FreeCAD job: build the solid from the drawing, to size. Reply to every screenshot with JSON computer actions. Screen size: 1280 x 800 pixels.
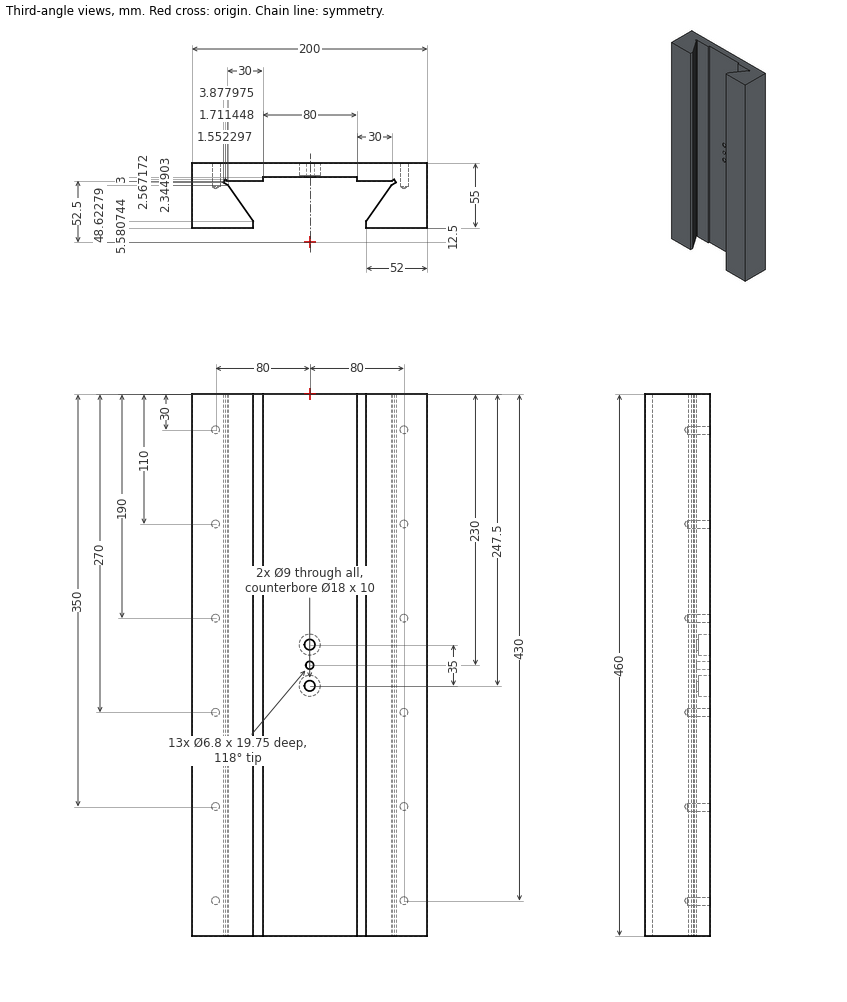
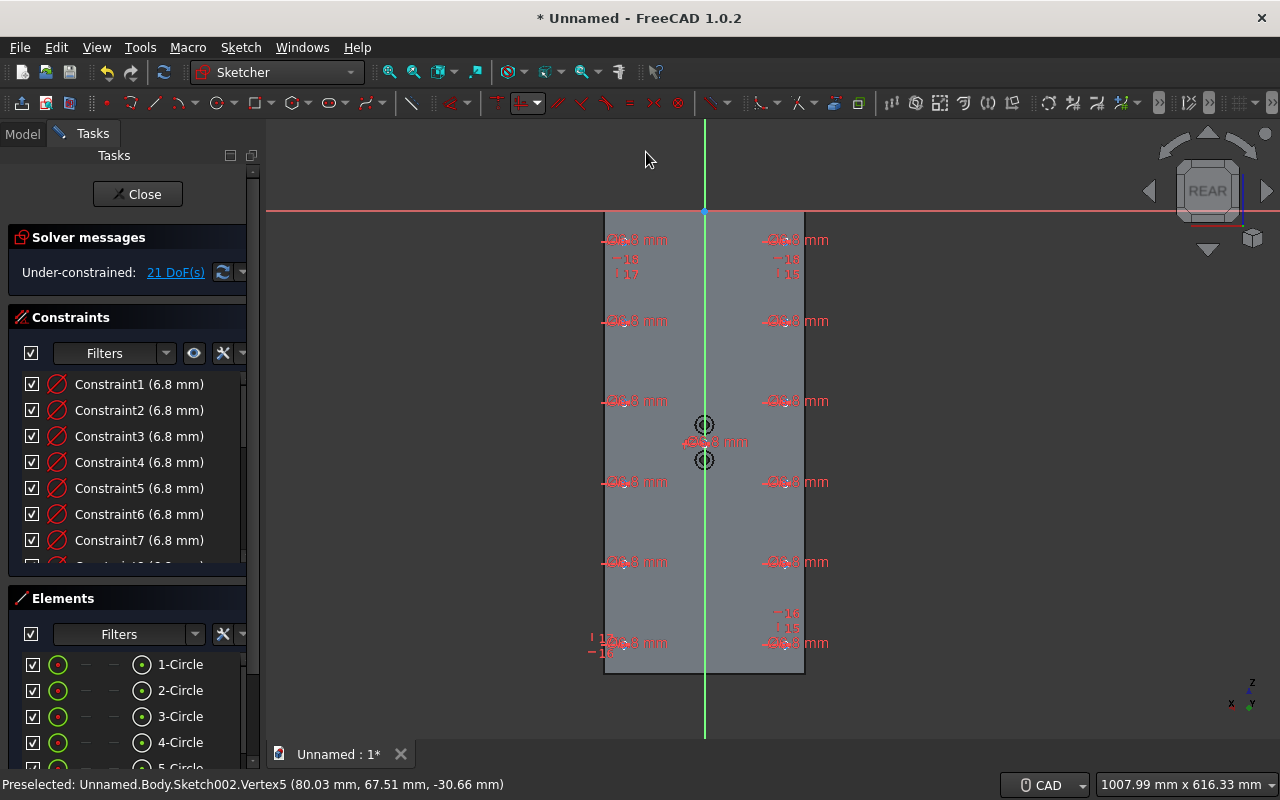
{"action": "left_click", "coordinate": [785, 645]}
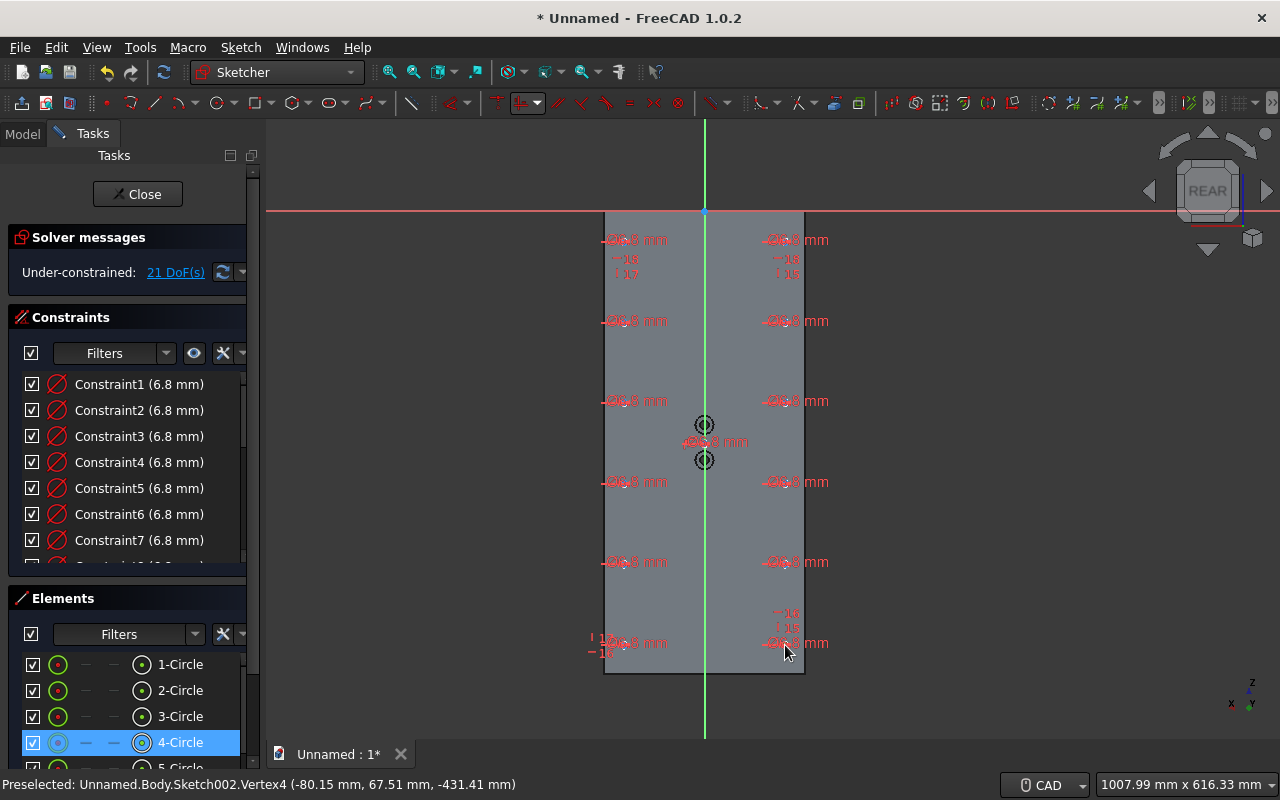
{"action": "left_click", "coordinate": [785, 564]}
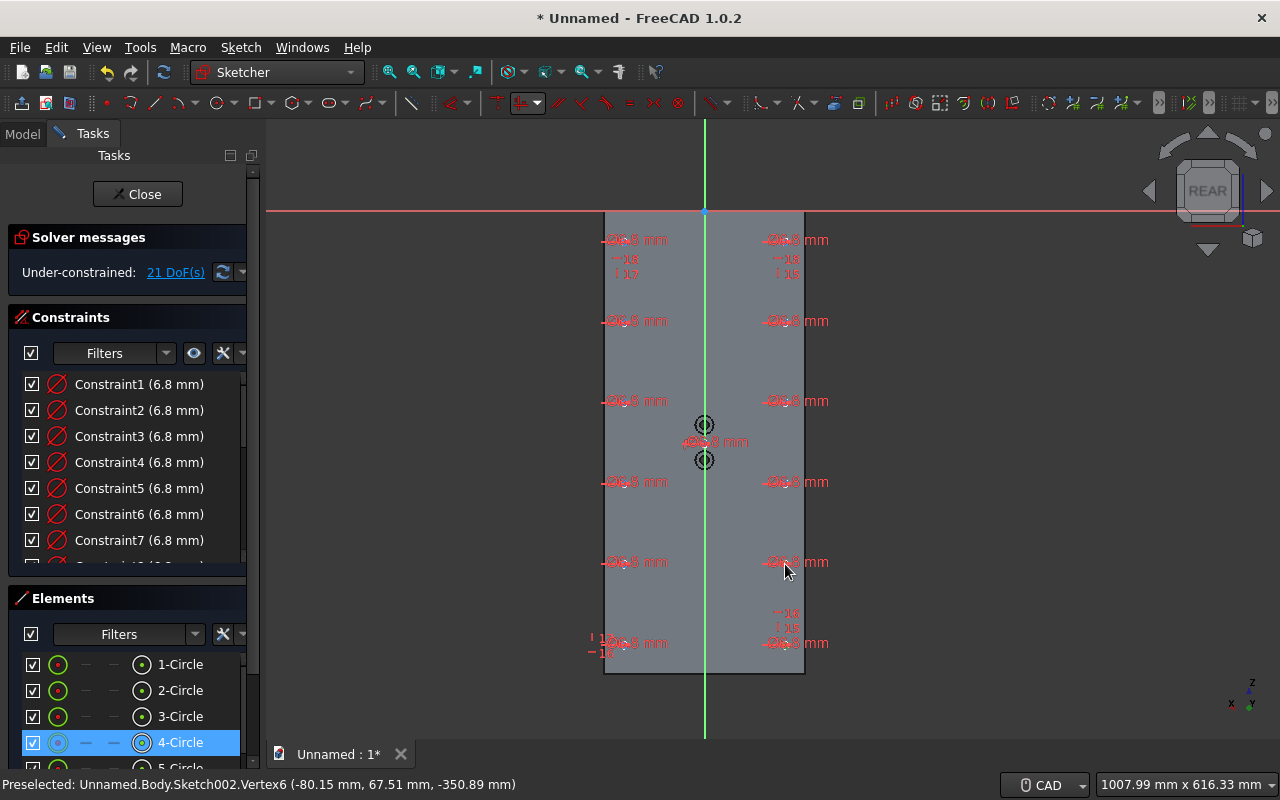
{"action": "key", "text": "v"}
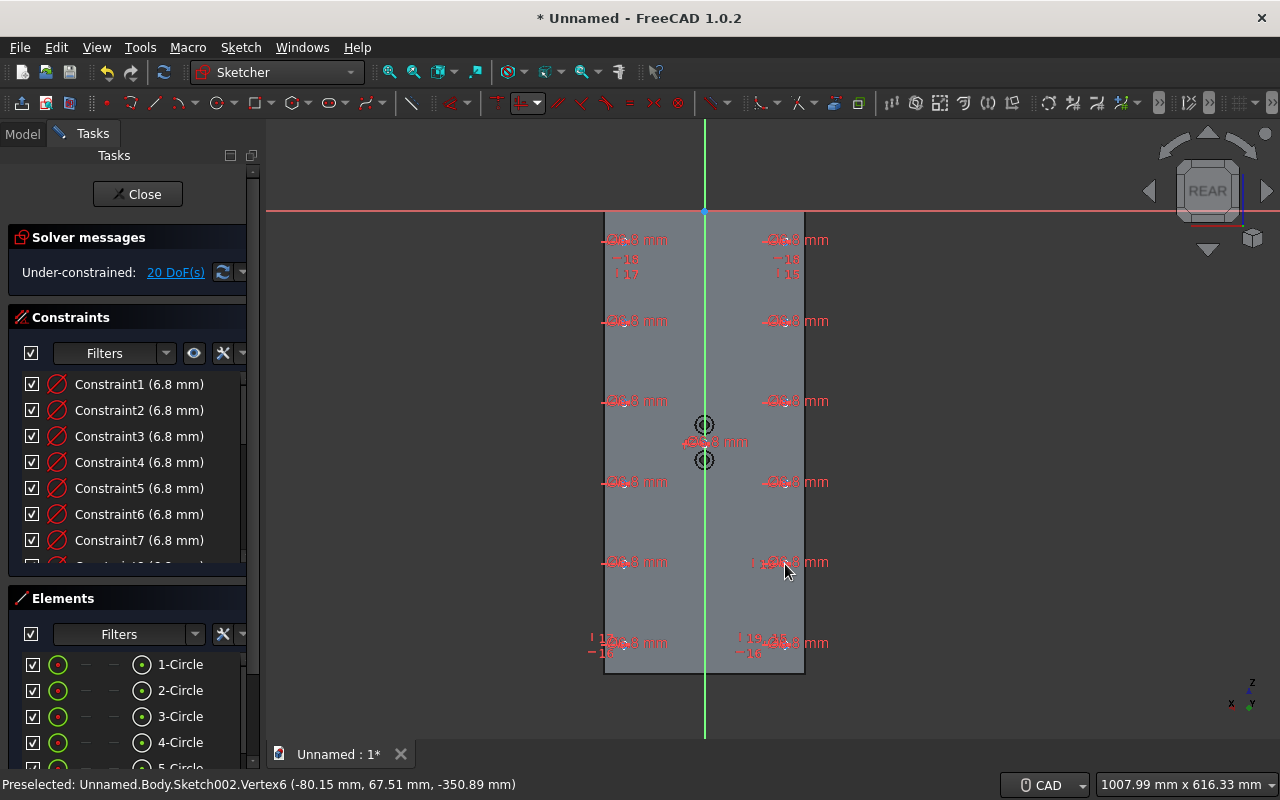
{"action": "left_click", "coordinate": [624, 645]}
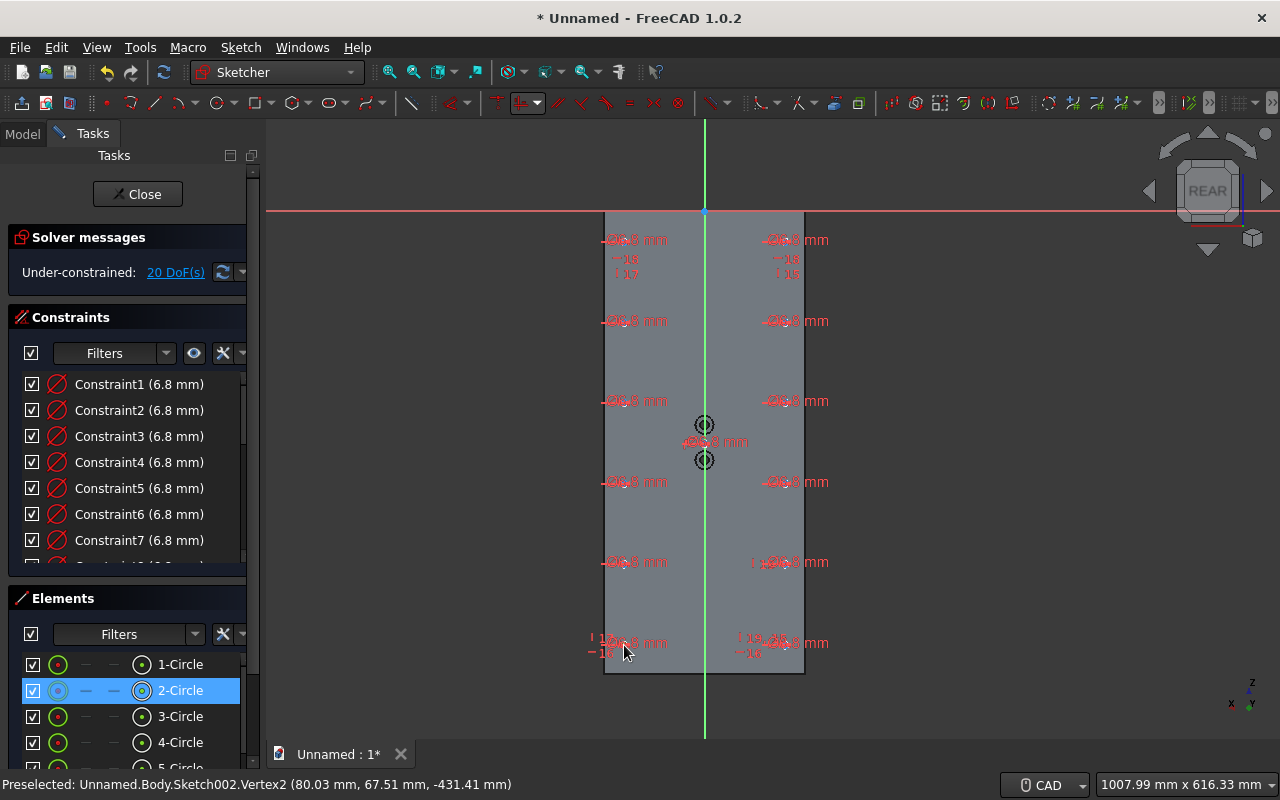
{"action": "left_click", "coordinate": [624, 564]}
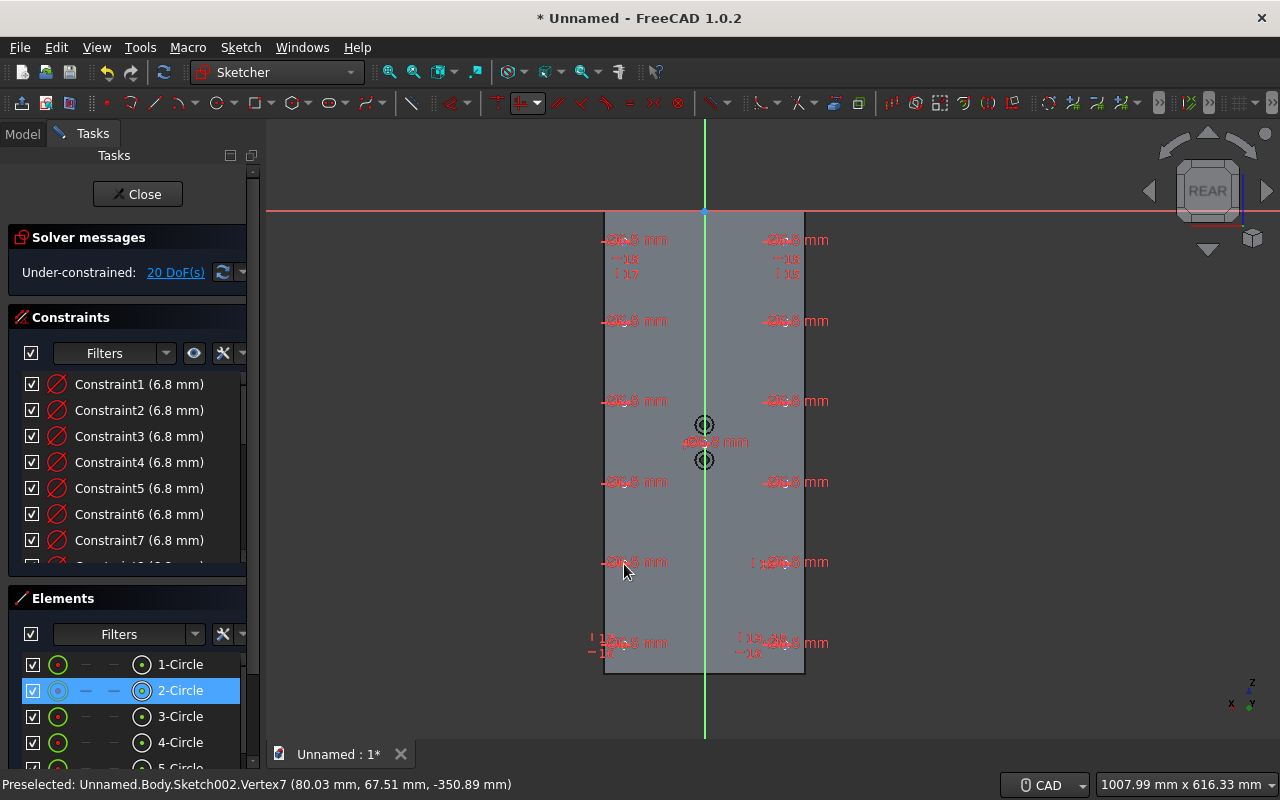
{"action": "left_click", "coordinate": [540, 104]}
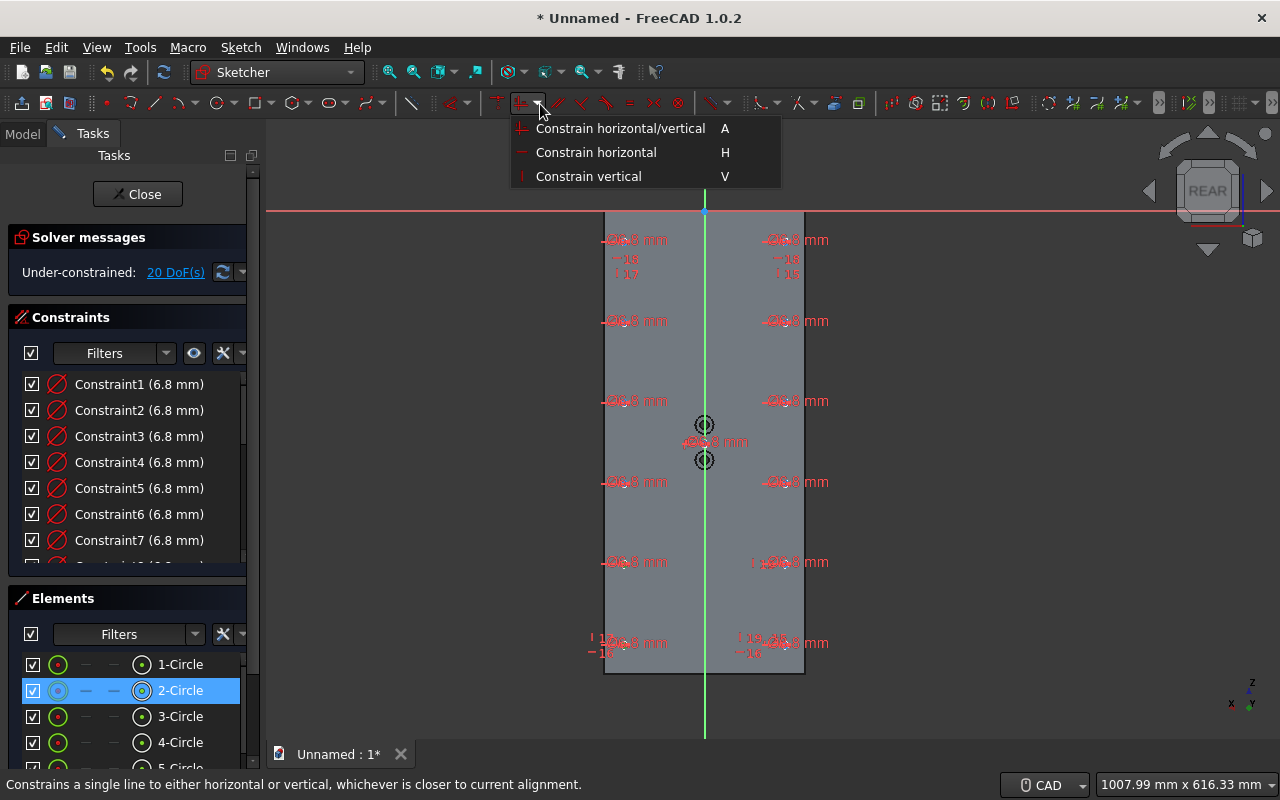
{"action": "left_click", "coordinate": [646, 176]}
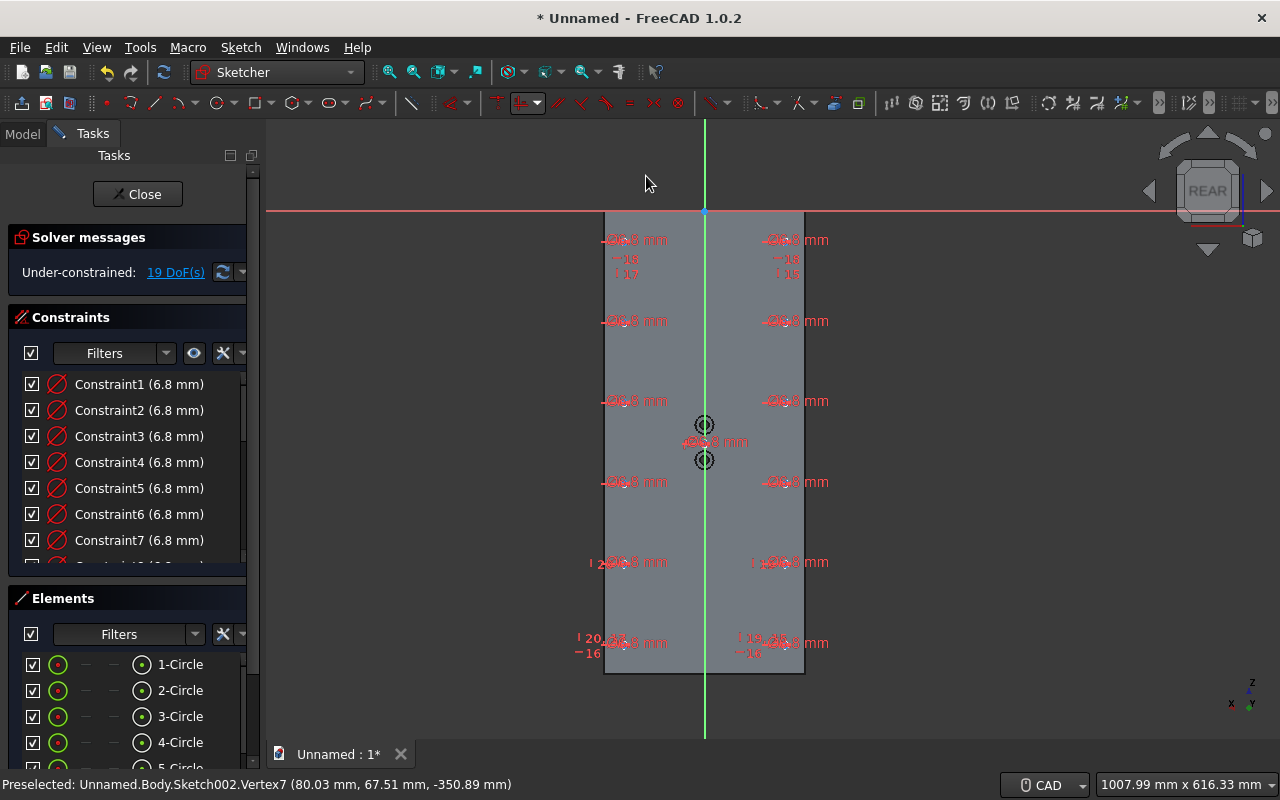
{"action": "left_click", "coordinate": [785, 564]}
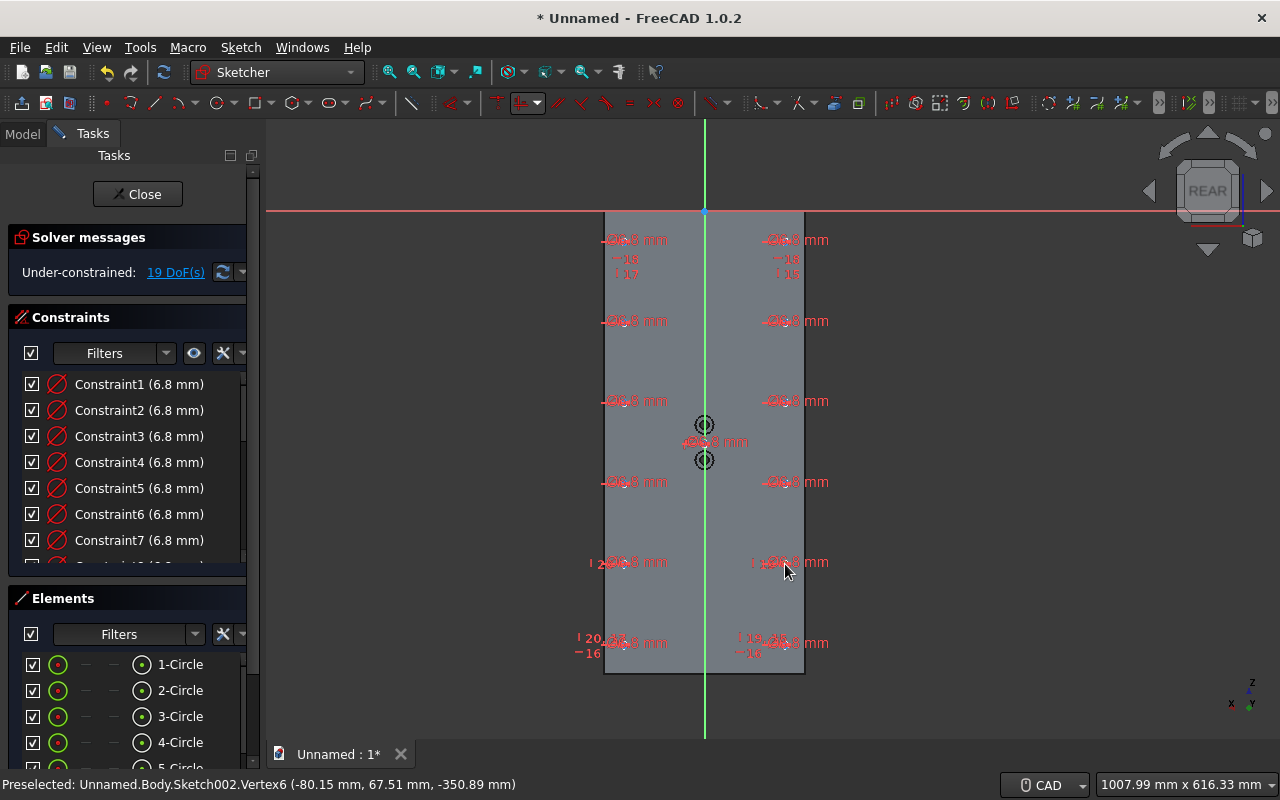
{"action": "left_click", "coordinate": [624, 564]}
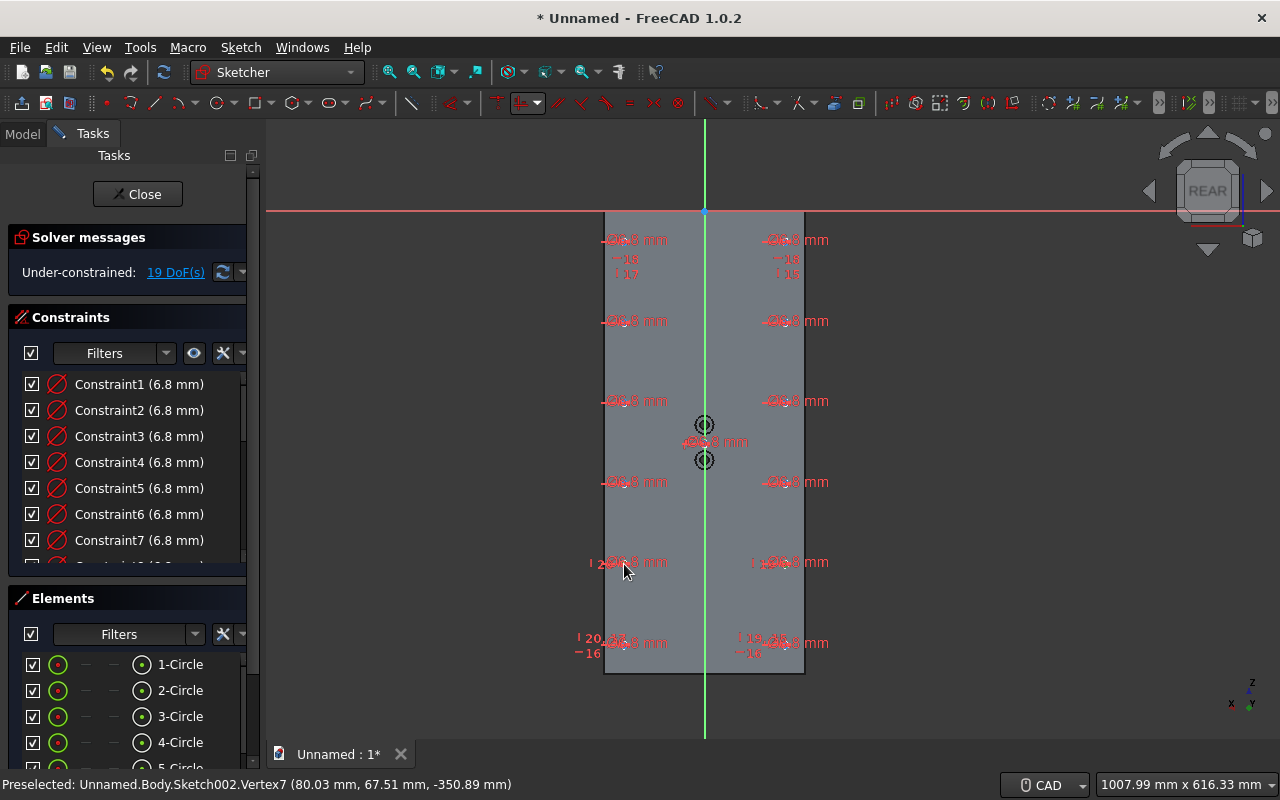
{"action": "key", "text": "h"}